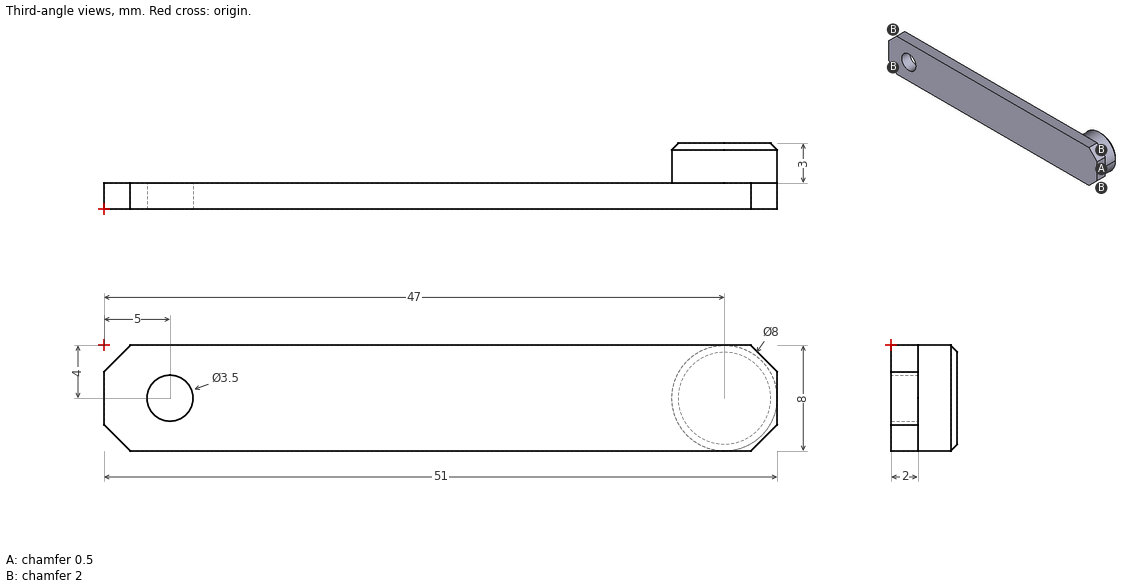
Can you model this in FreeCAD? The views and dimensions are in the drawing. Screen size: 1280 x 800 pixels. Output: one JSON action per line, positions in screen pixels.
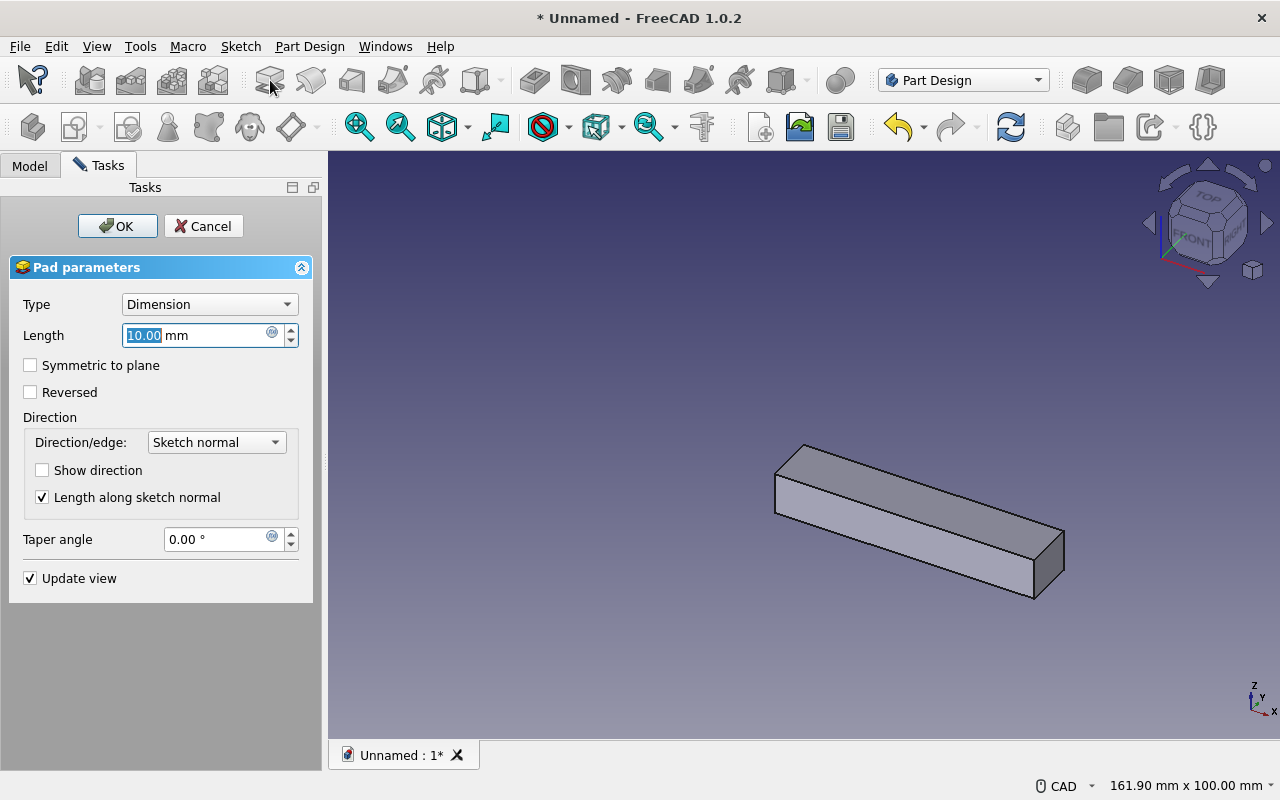
{"action": "type", "text": "2"}
{"action": "key", "text": "Tab"}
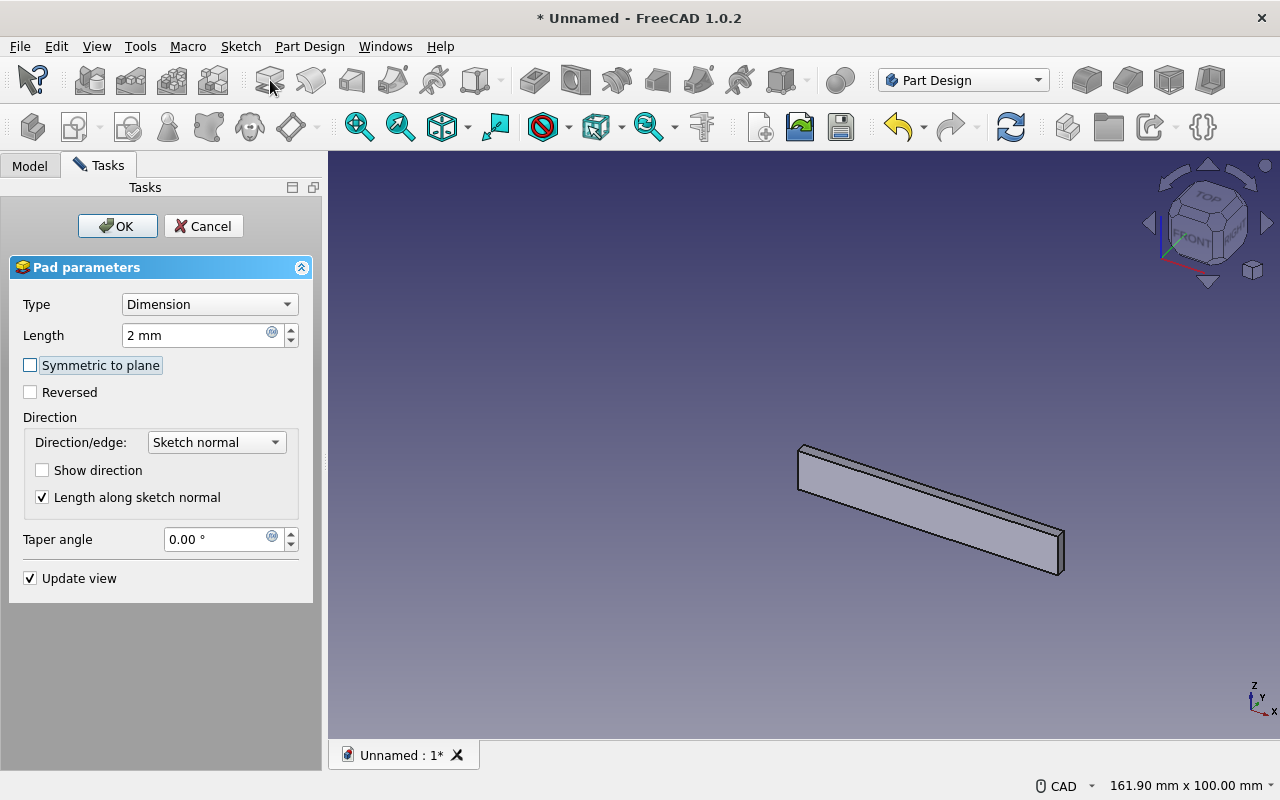
{"action": "left_click", "coordinate": [31, 392]}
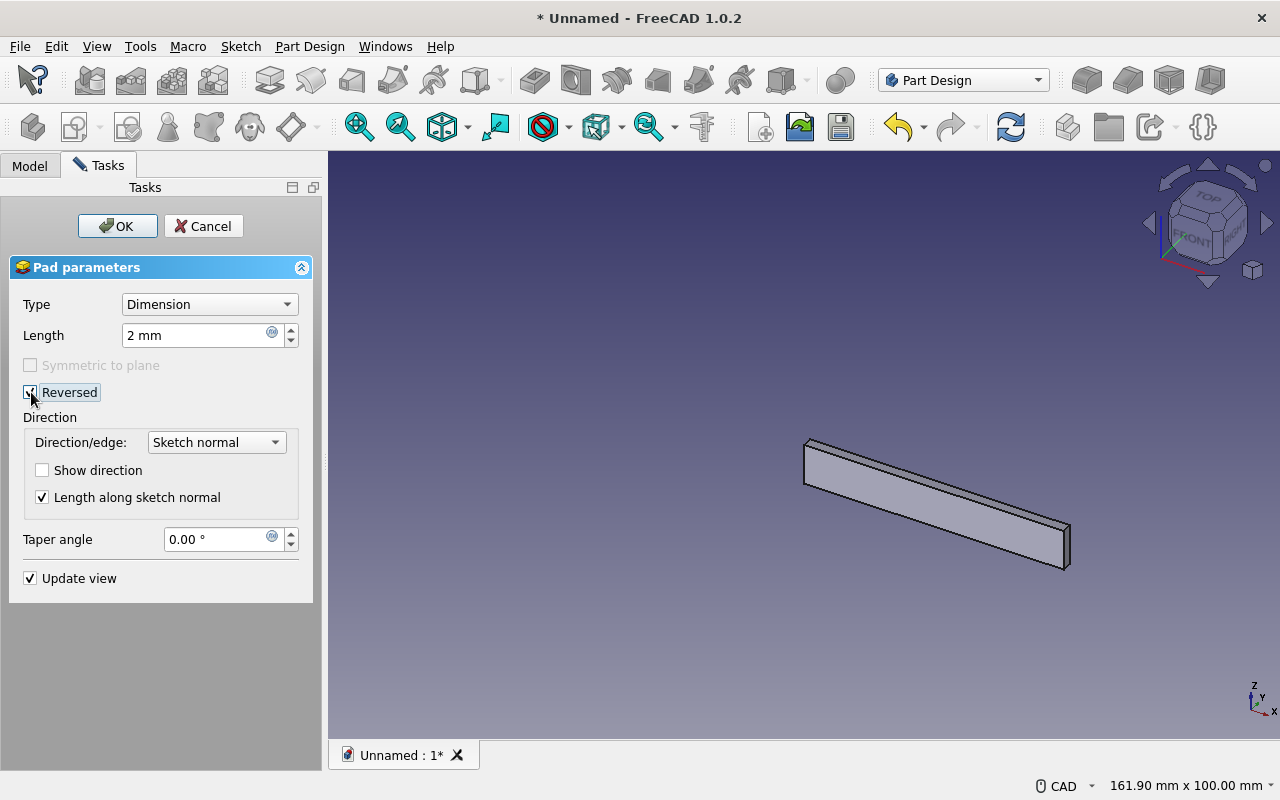
{"action": "left_click", "coordinate": [118, 226]}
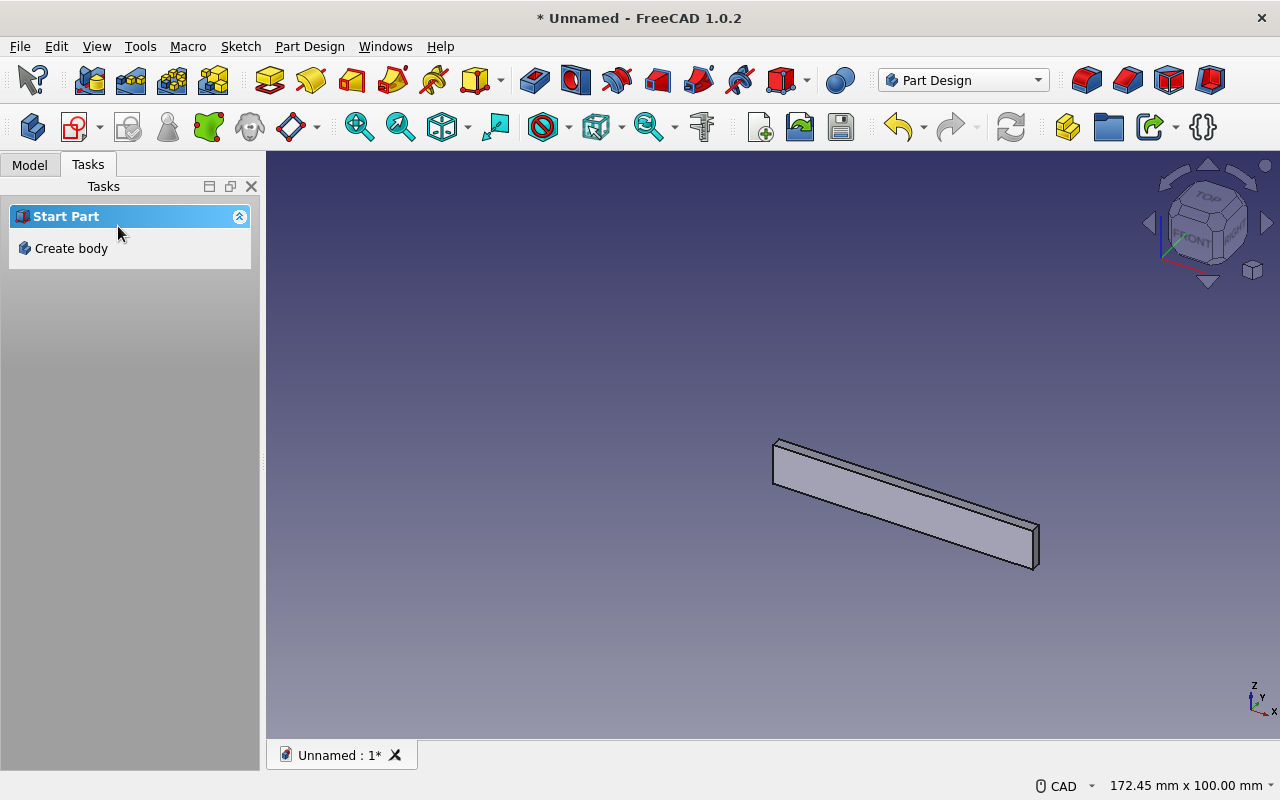
{"action": "key", "text": "v f"}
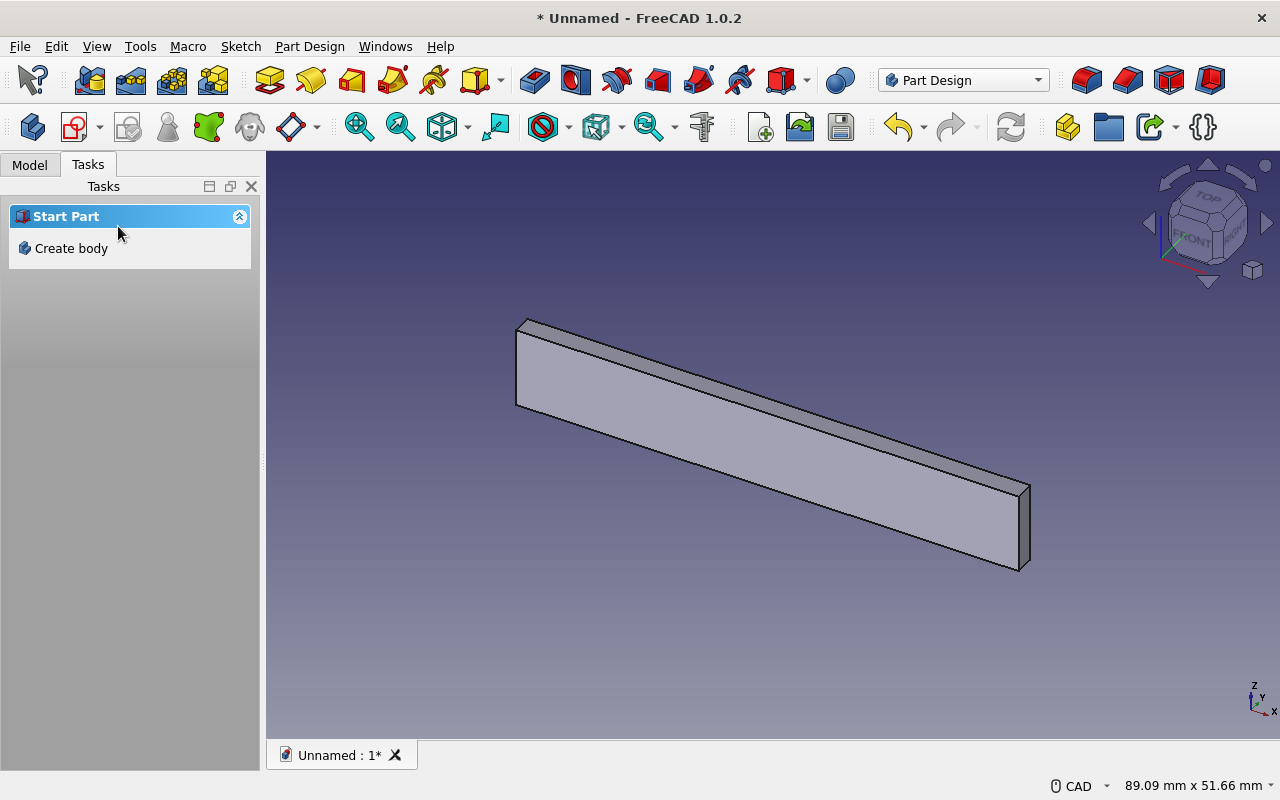
{"action": "key", "text": "4"}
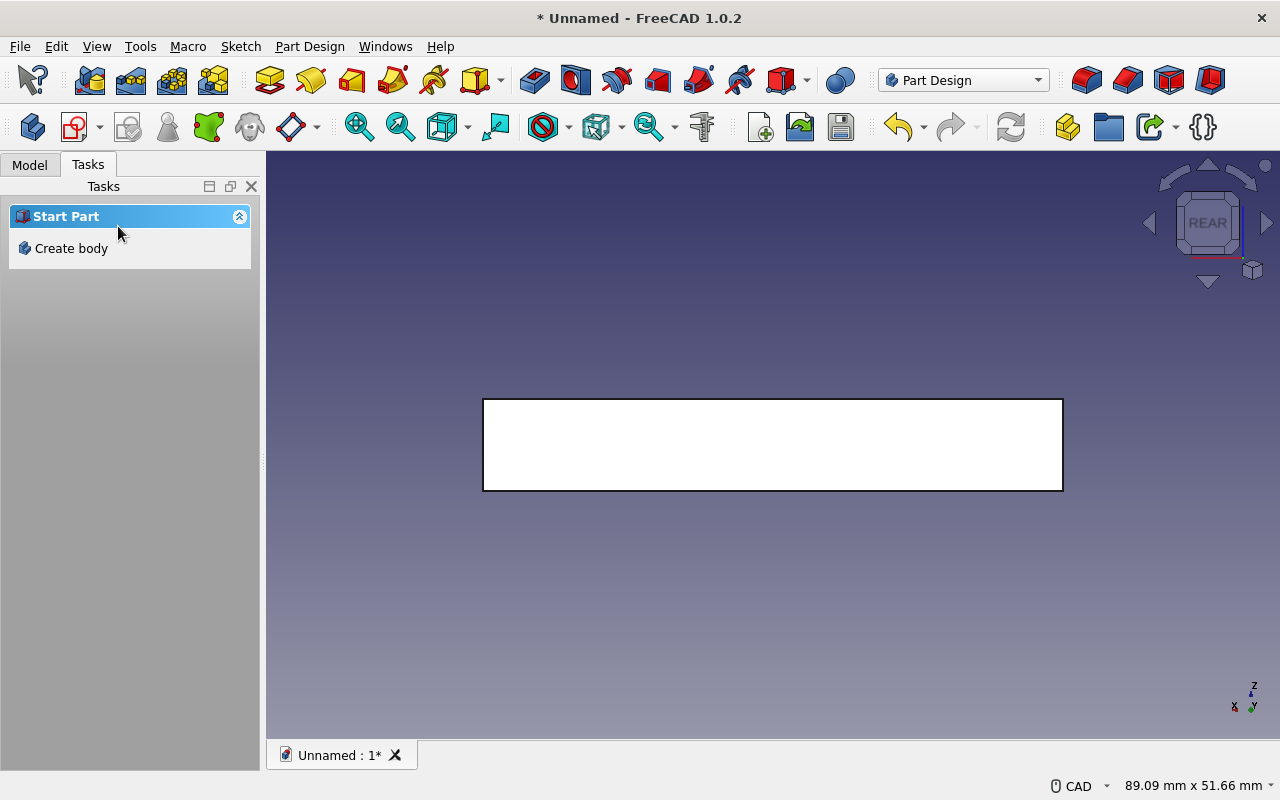
{"action": "left_click", "coordinate": [607, 444]}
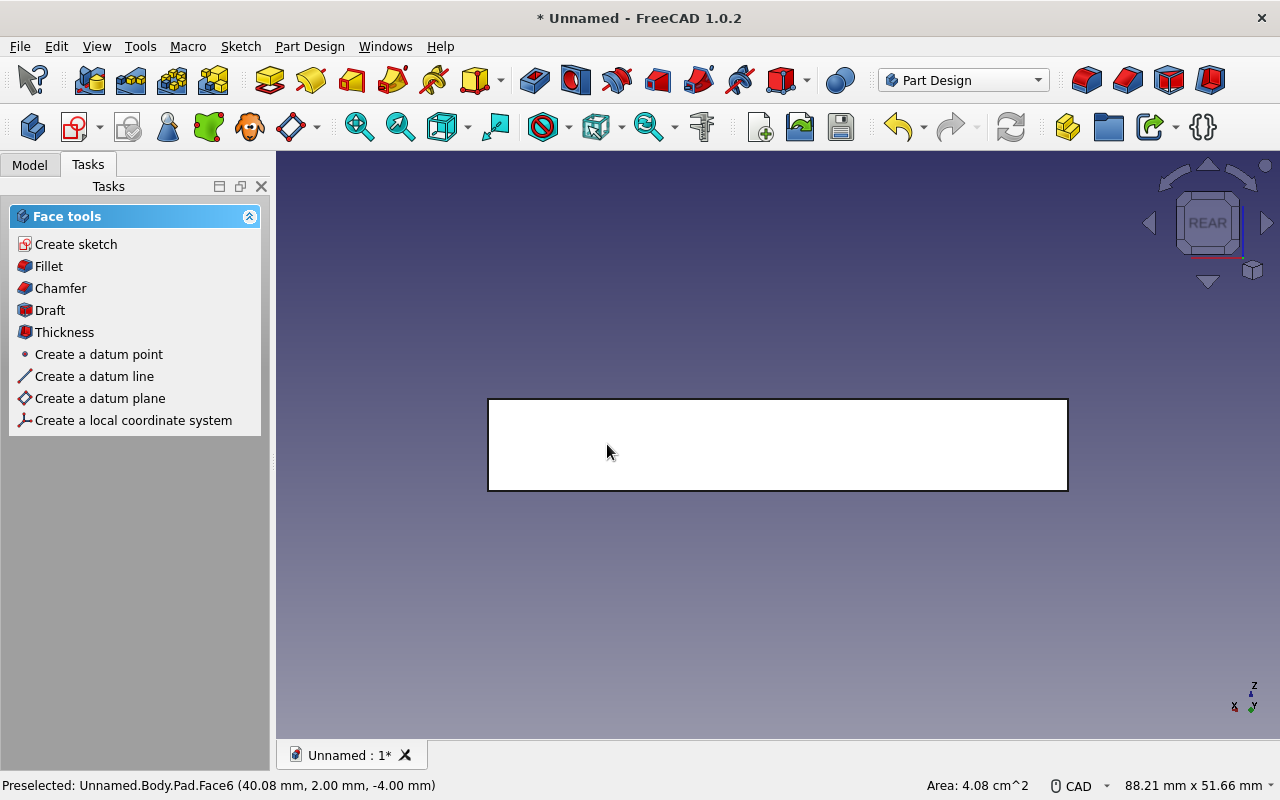
{"action": "left_click", "coordinate": [74, 128]}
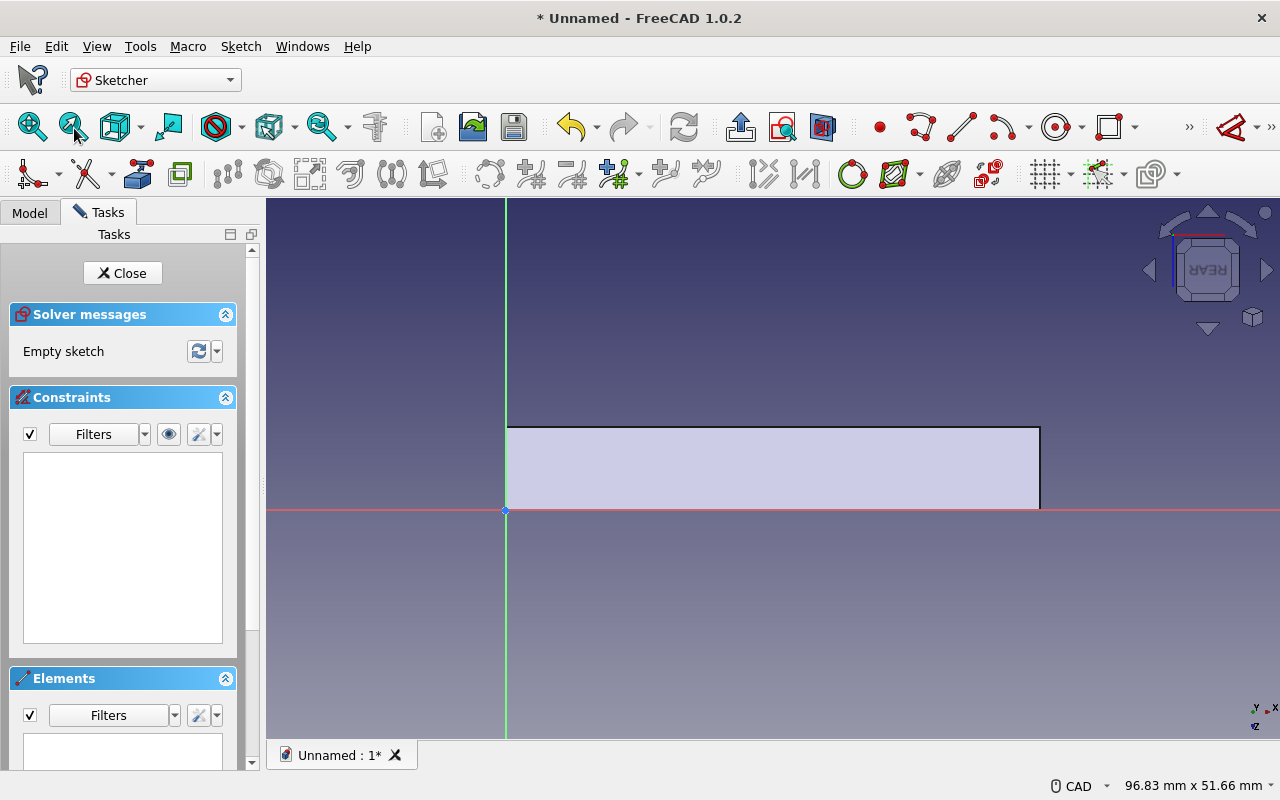
{"action": "scroll", "coordinate": [509, 483], "scroll_direction": "up", "scroll_amount": 9}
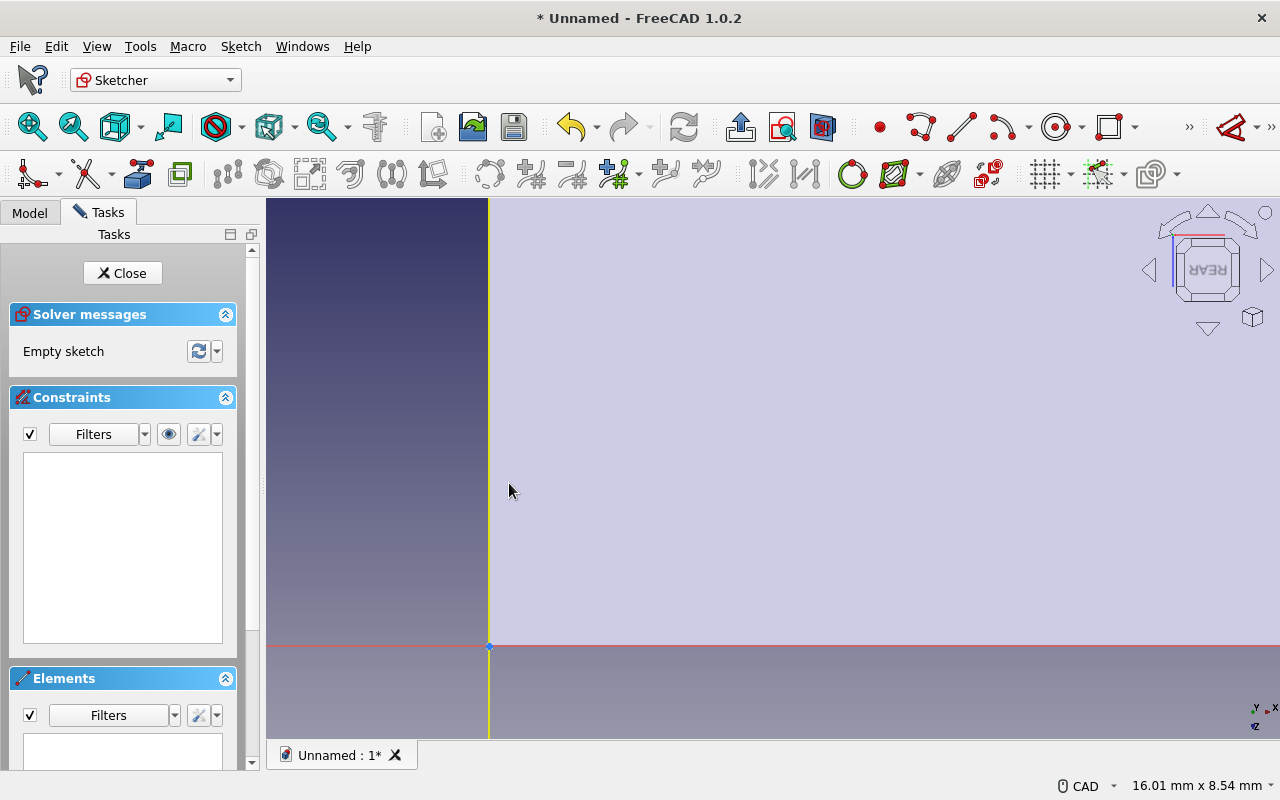
{"action": "left_click", "coordinate": [1056, 128]}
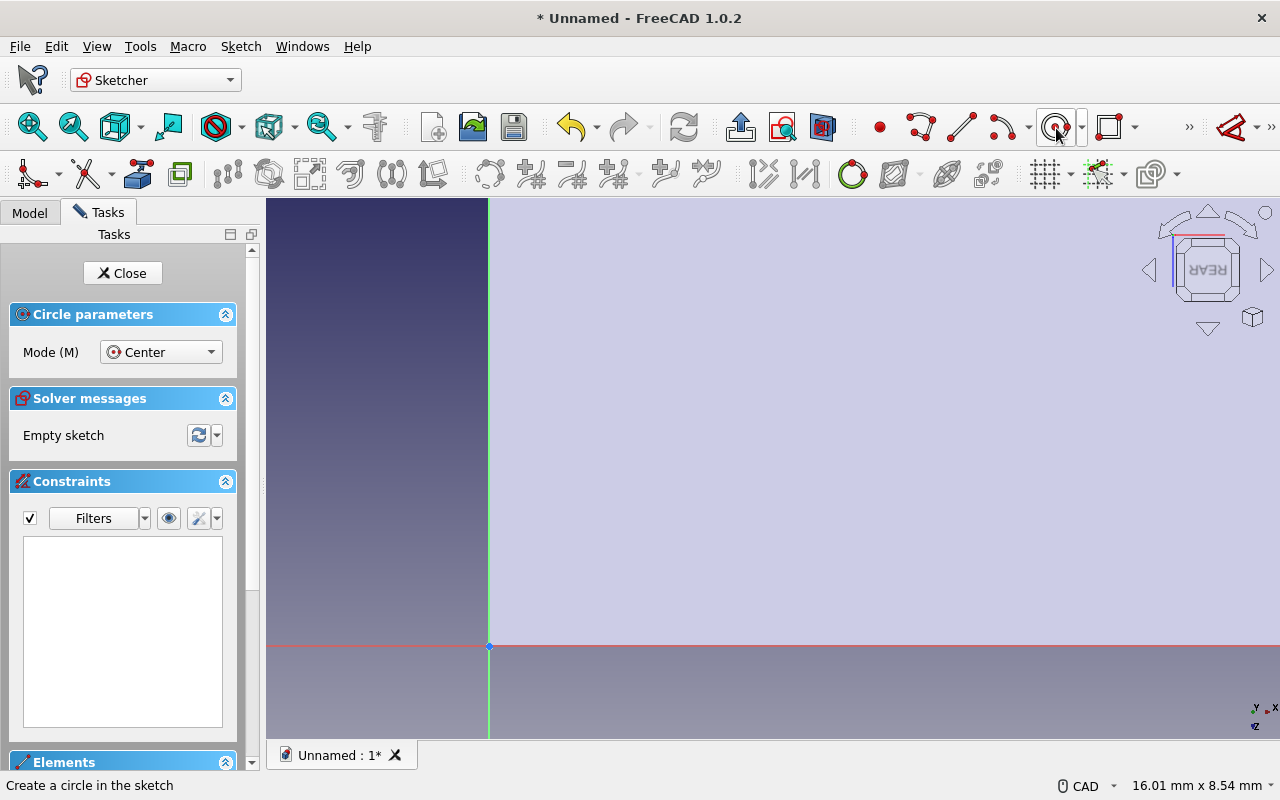
{"action": "left_click", "coordinate": [806, 393]}
{"action": "mouse_move", "coordinate": [885, 314]}